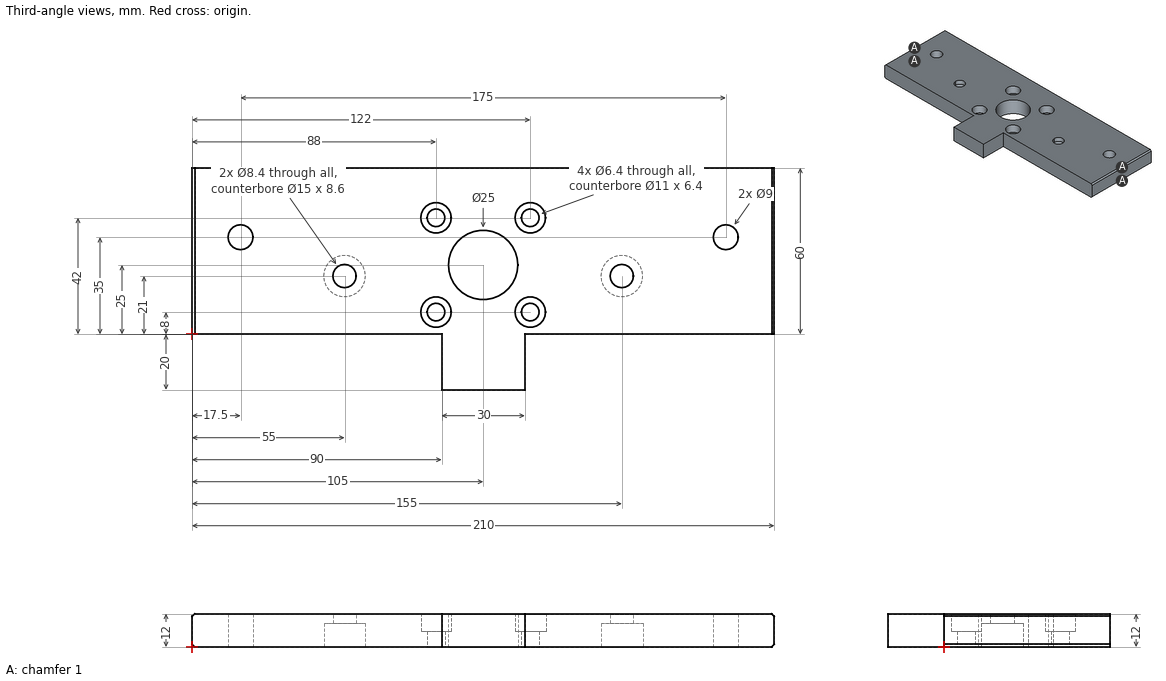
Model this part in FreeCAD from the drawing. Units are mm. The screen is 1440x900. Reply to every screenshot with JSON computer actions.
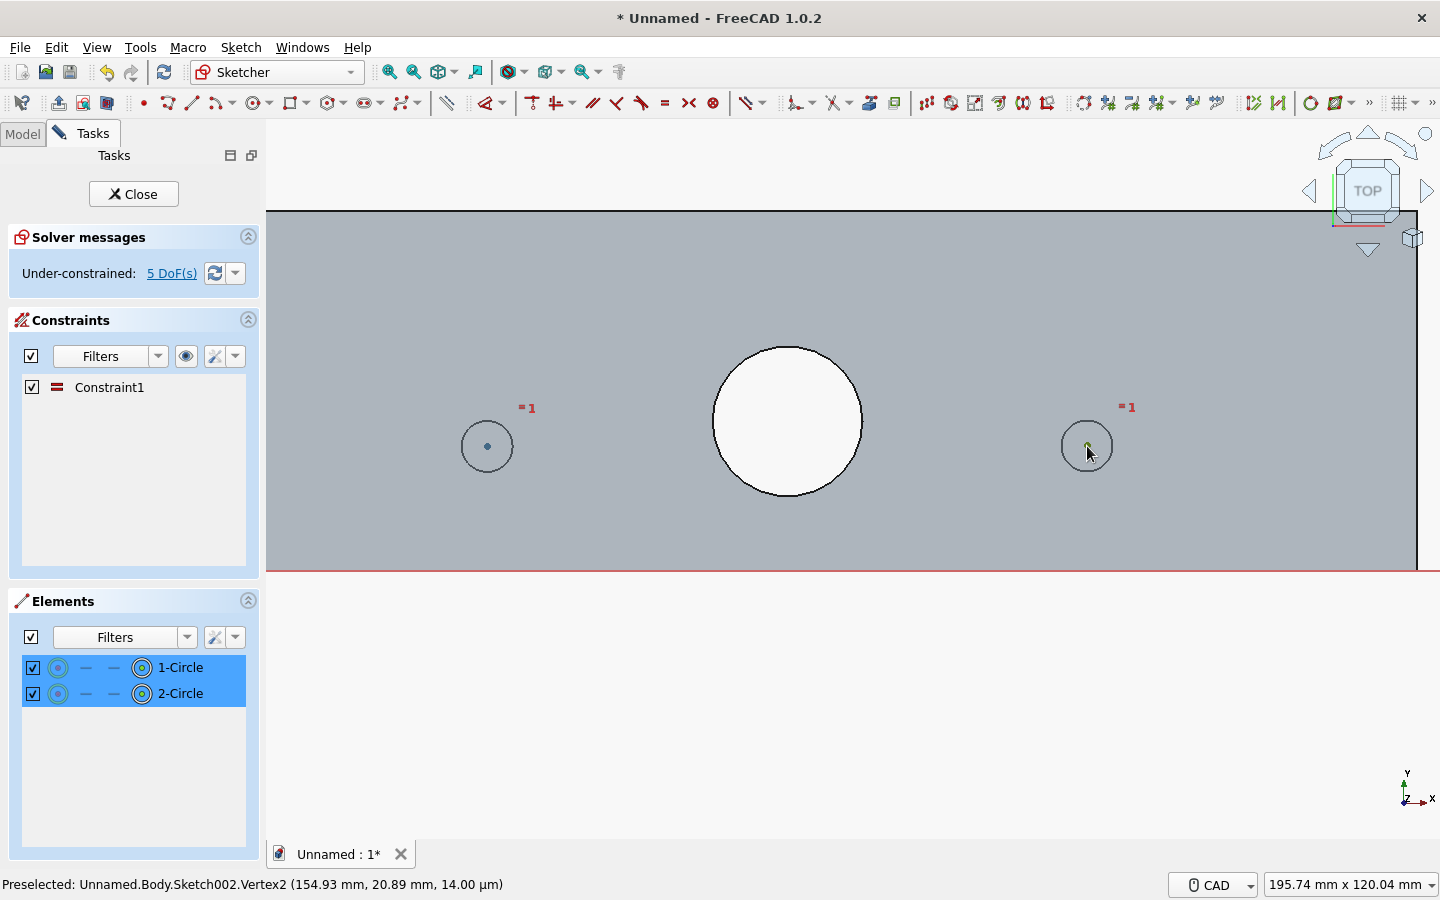
{"action": "key", "text": "h"}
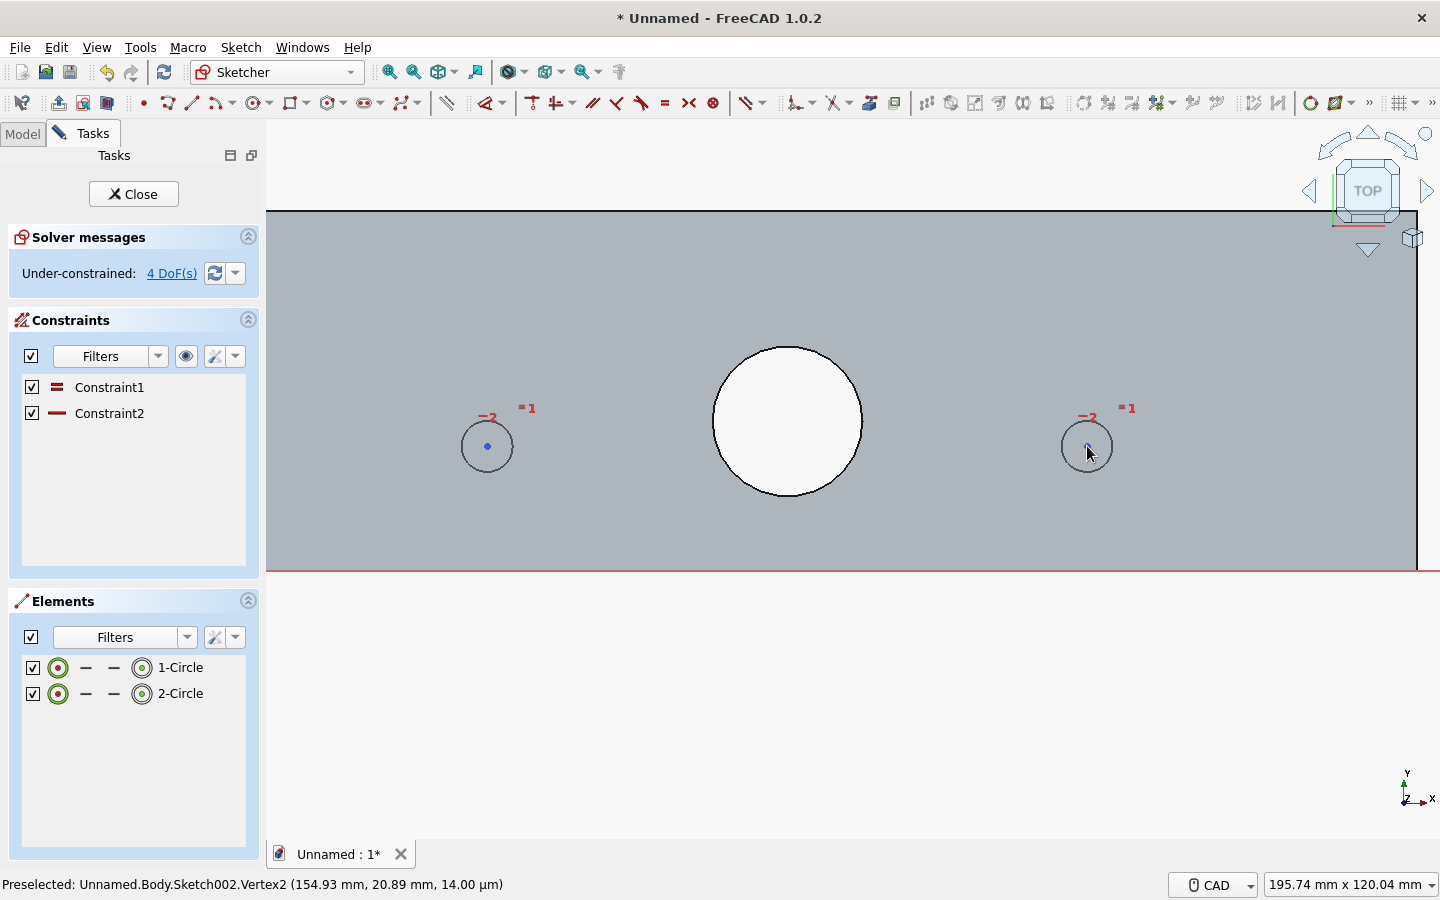
{"action": "key", "text": "d"}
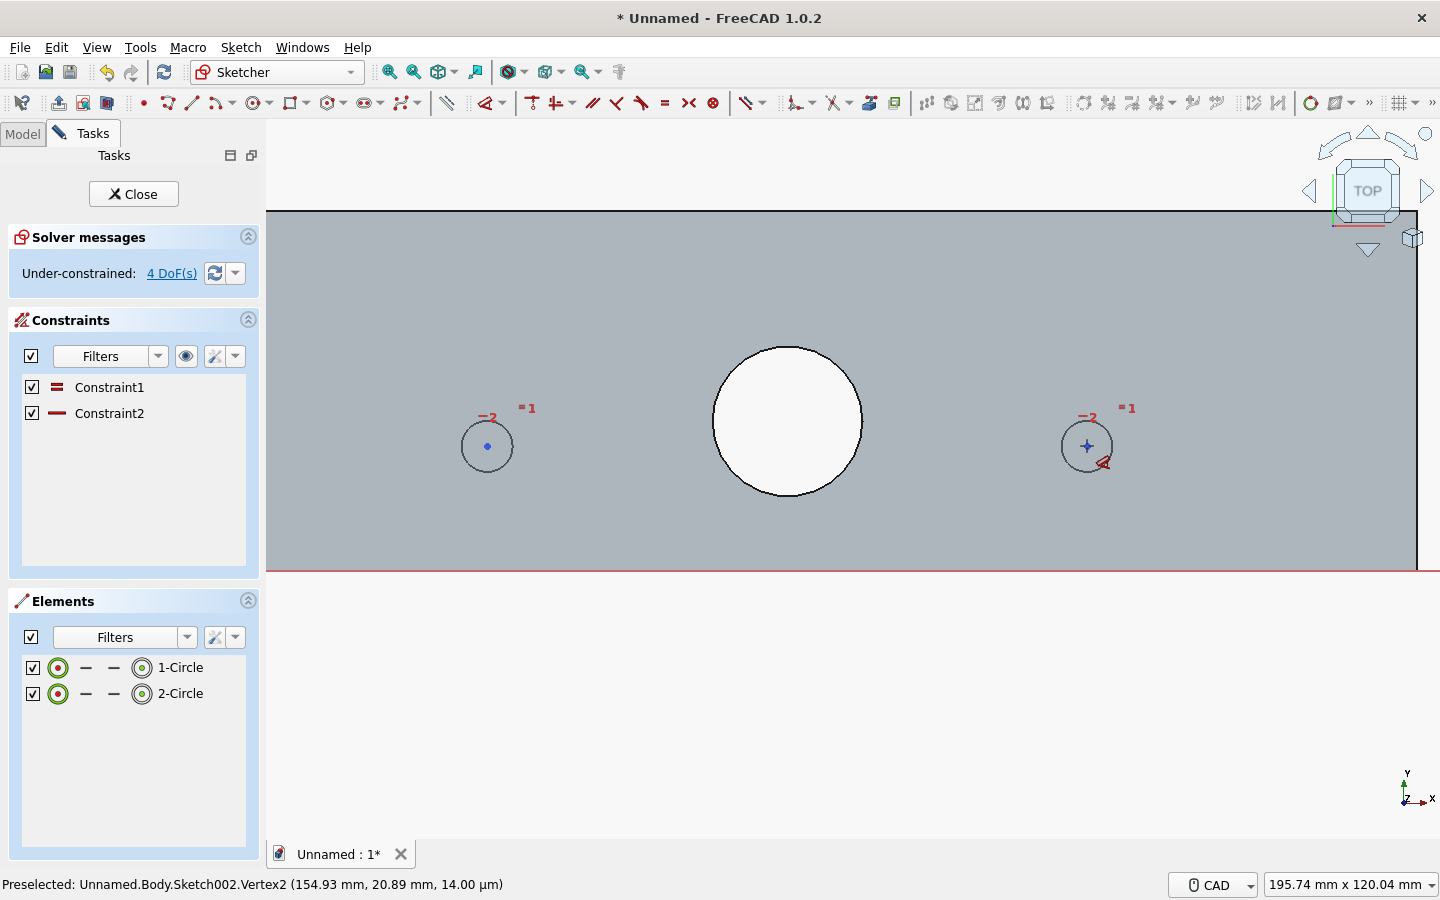
{"action": "left_click", "coordinate": [505, 428]}
{"action": "left_click", "coordinate": [527, 405]}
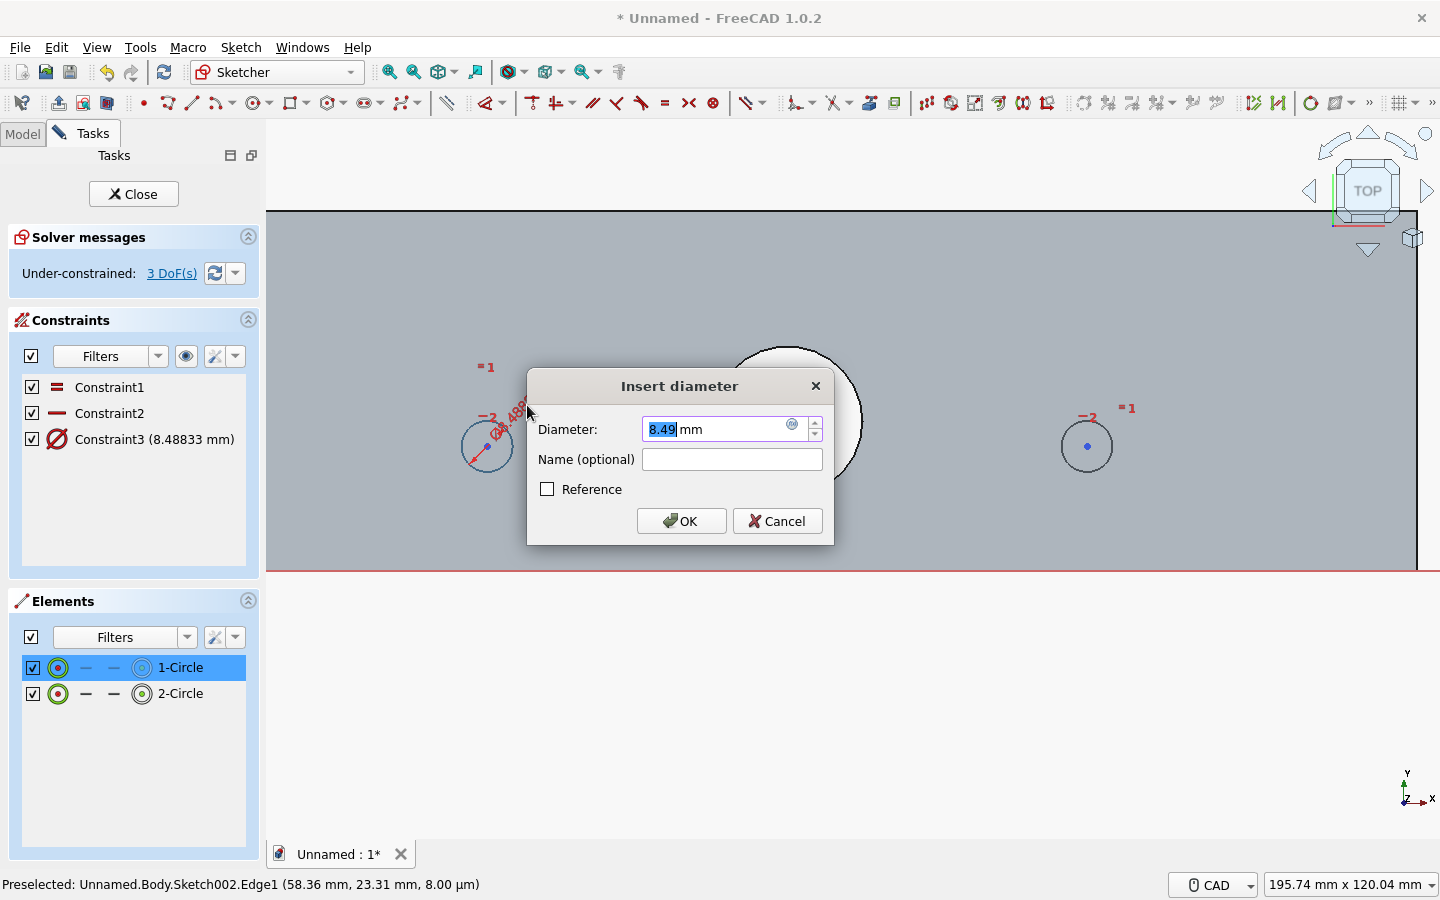
{"action": "type", "text": "8.4"}
{"action": "key", "text": "Return"}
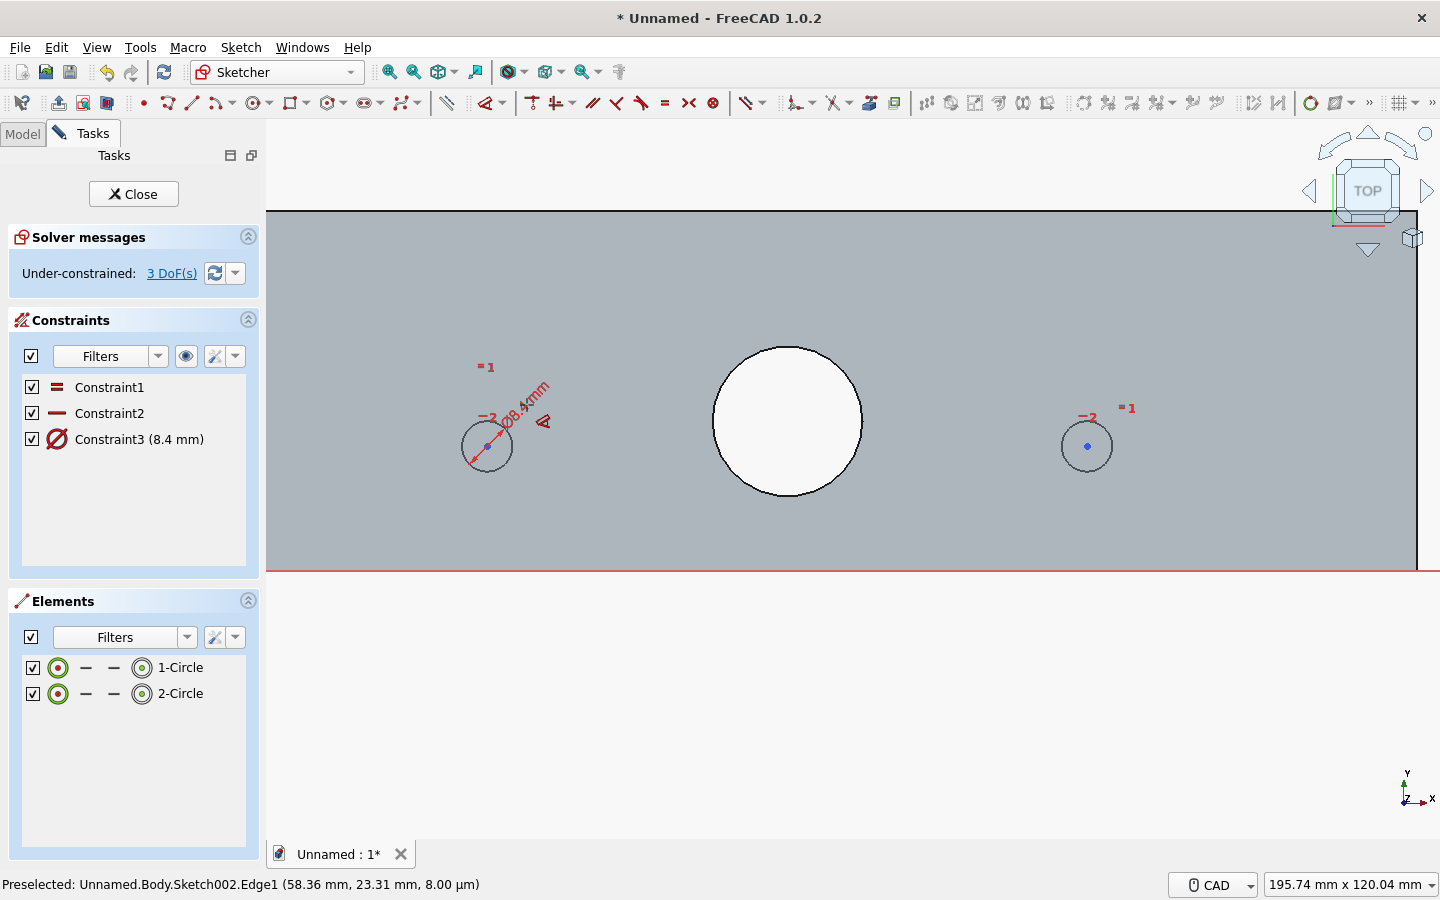
{"action": "left_click", "coordinate": [487, 446]}
{"action": "left_click", "coordinate": [391, 605]}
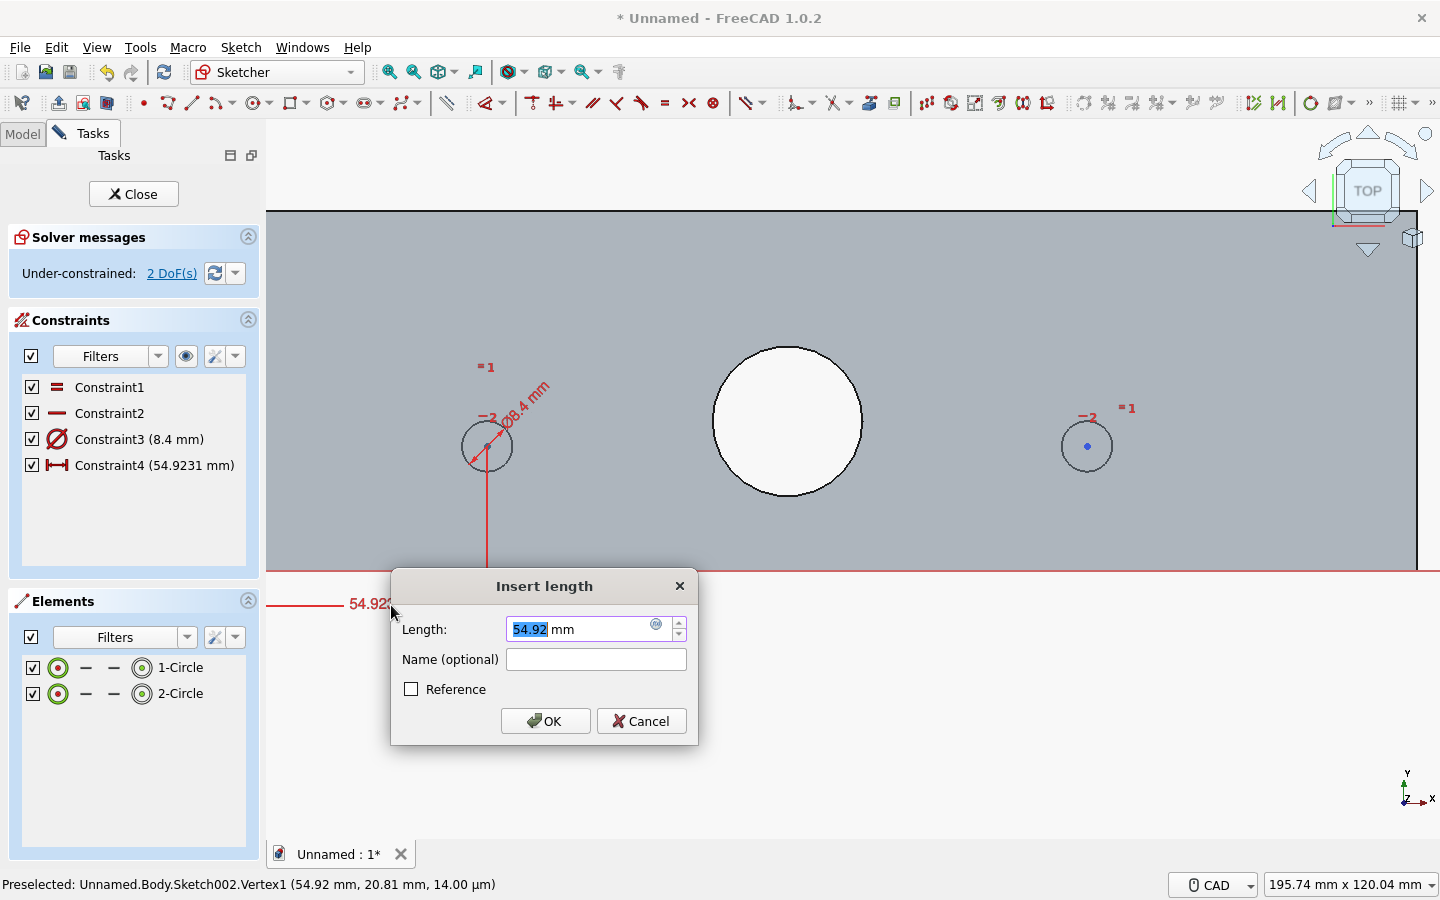
{"action": "type", "text": "55"}
{"action": "key", "text": "Return"}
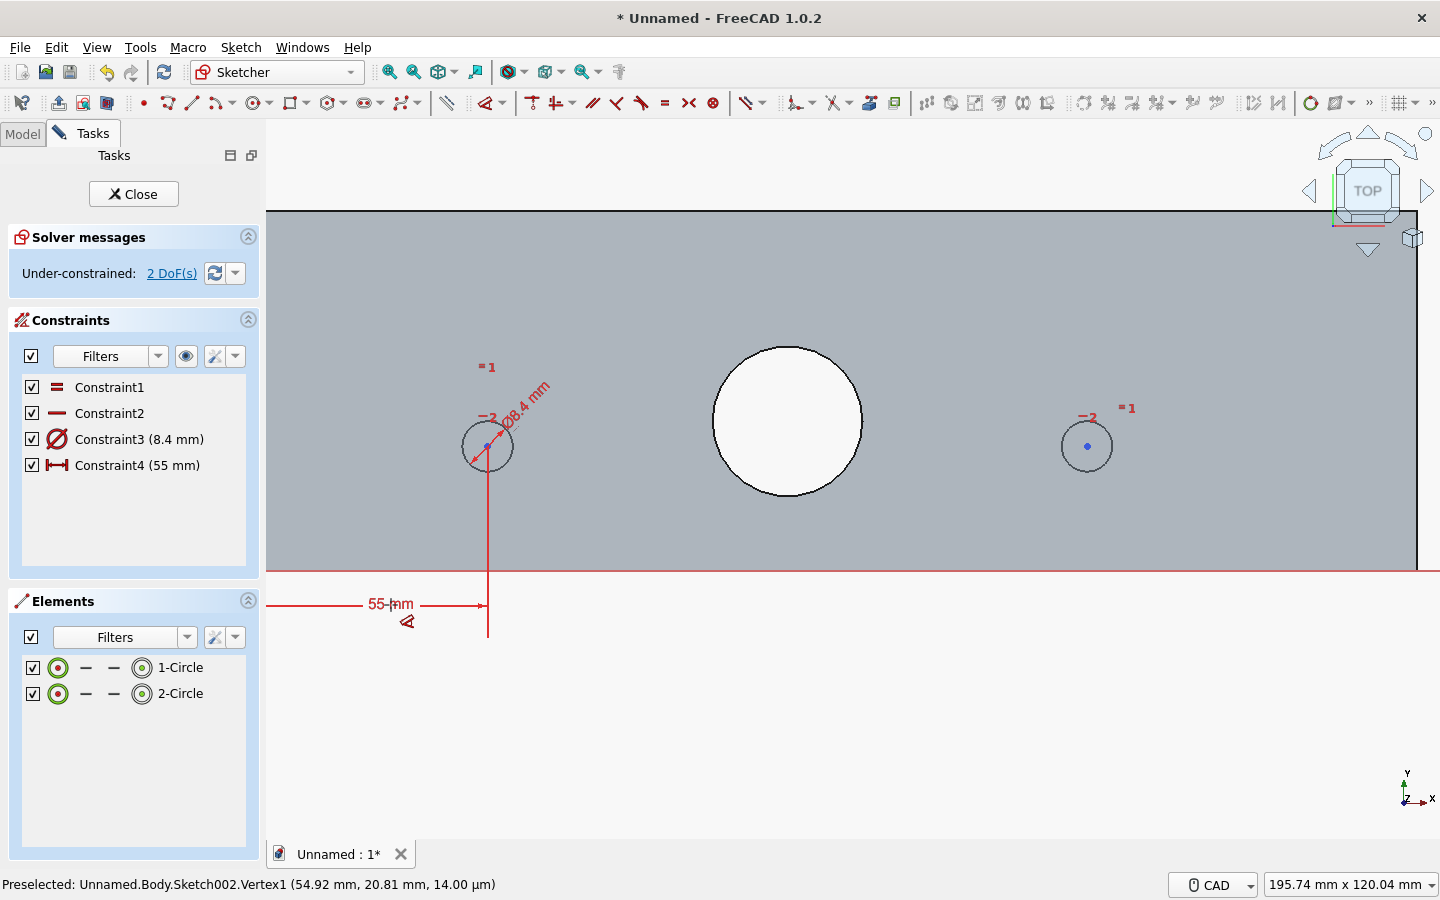
{"action": "left_click", "coordinate": [488, 446]}
{"action": "left_click", "coordinate": [522, 509]}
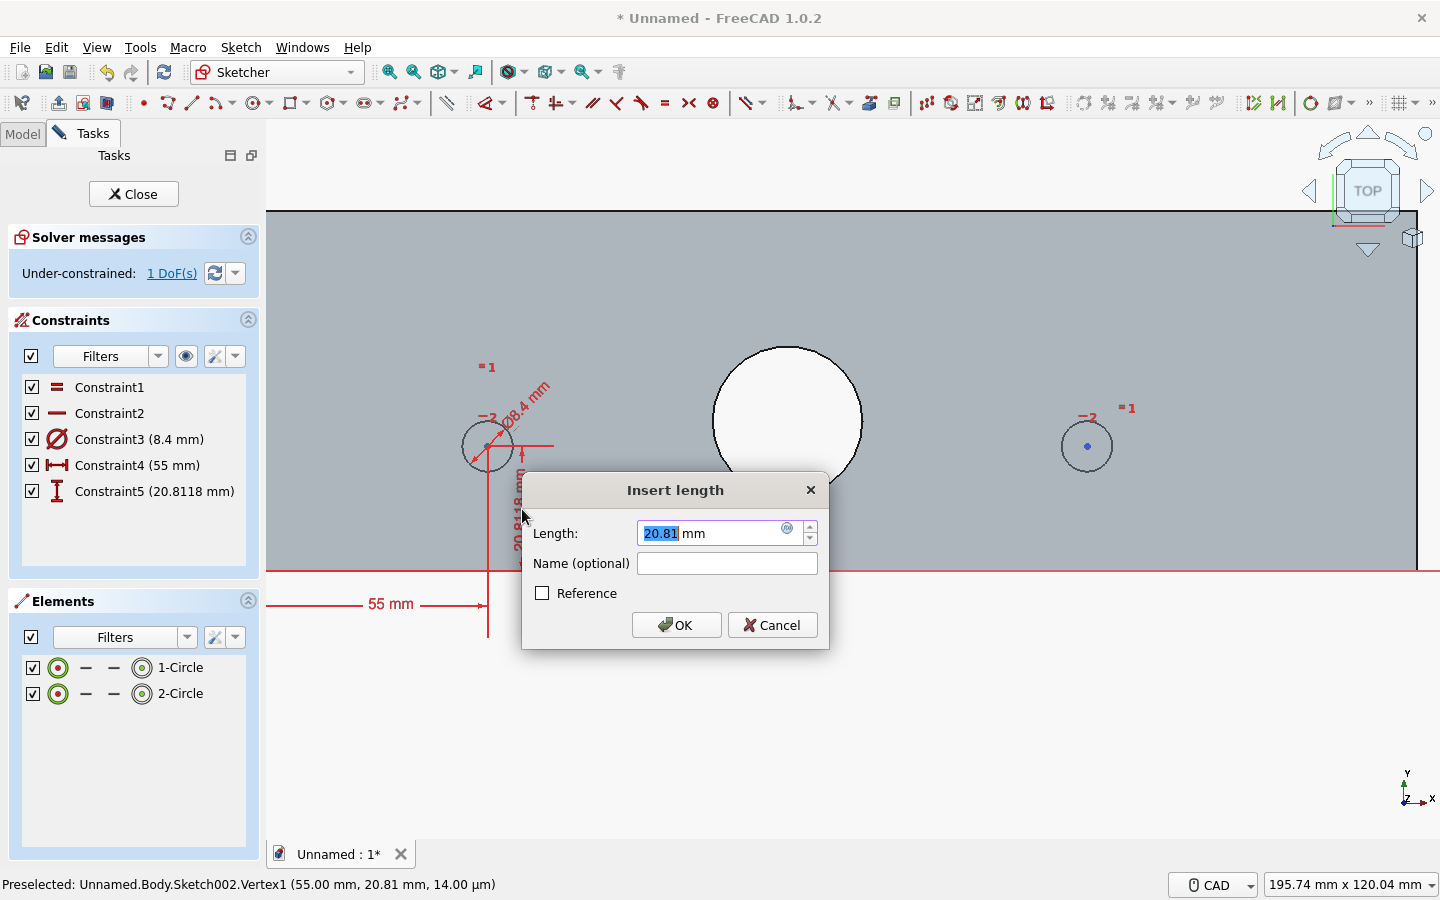
{"action": "type", "text": "21"}
{"action": "key", "text": "Return"}